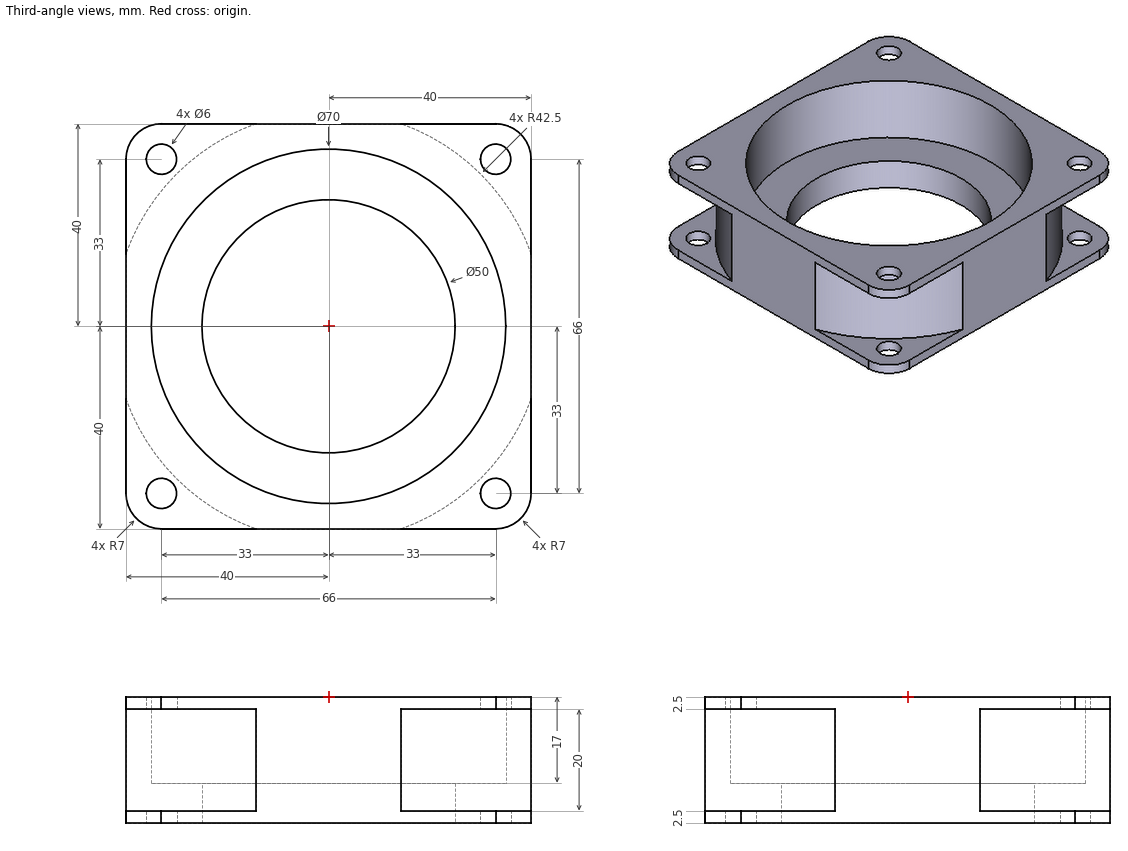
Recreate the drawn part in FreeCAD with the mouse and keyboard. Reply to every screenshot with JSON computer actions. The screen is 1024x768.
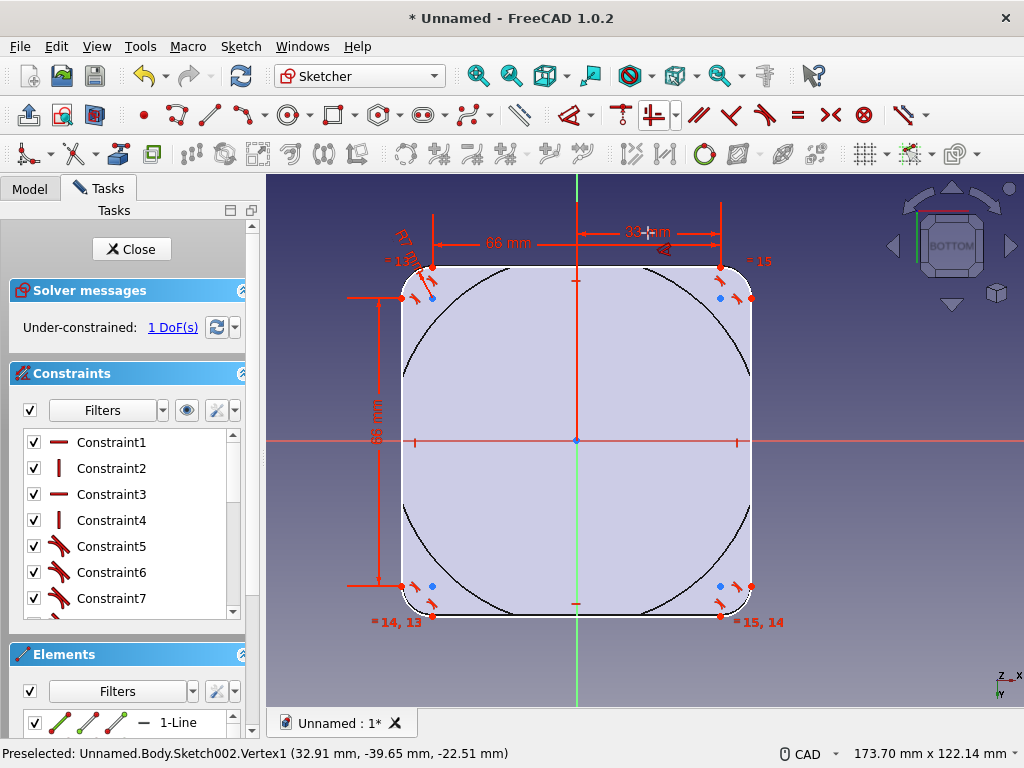
{"action": "left_click", "coordinate": [721, 267]}
{"action": "left_click", "coordinate": [543, 354]}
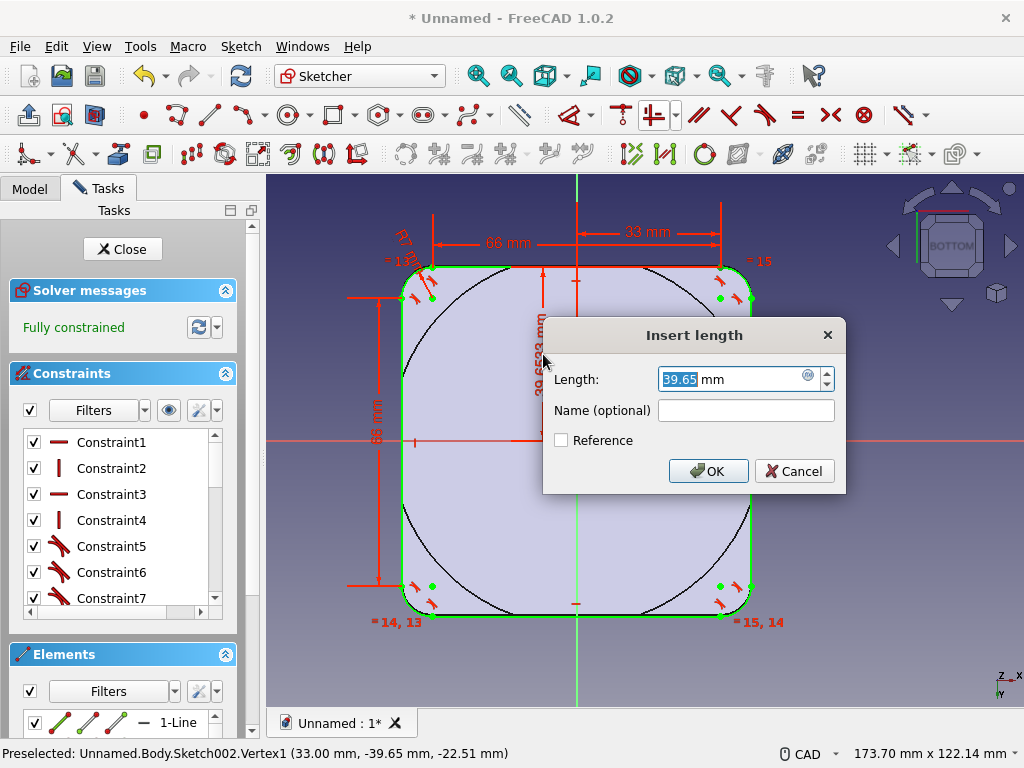
{"action": "type", "text": "40"}
{"action": "key", "text": "Return"}
{"action": "key", "text": "Escape"}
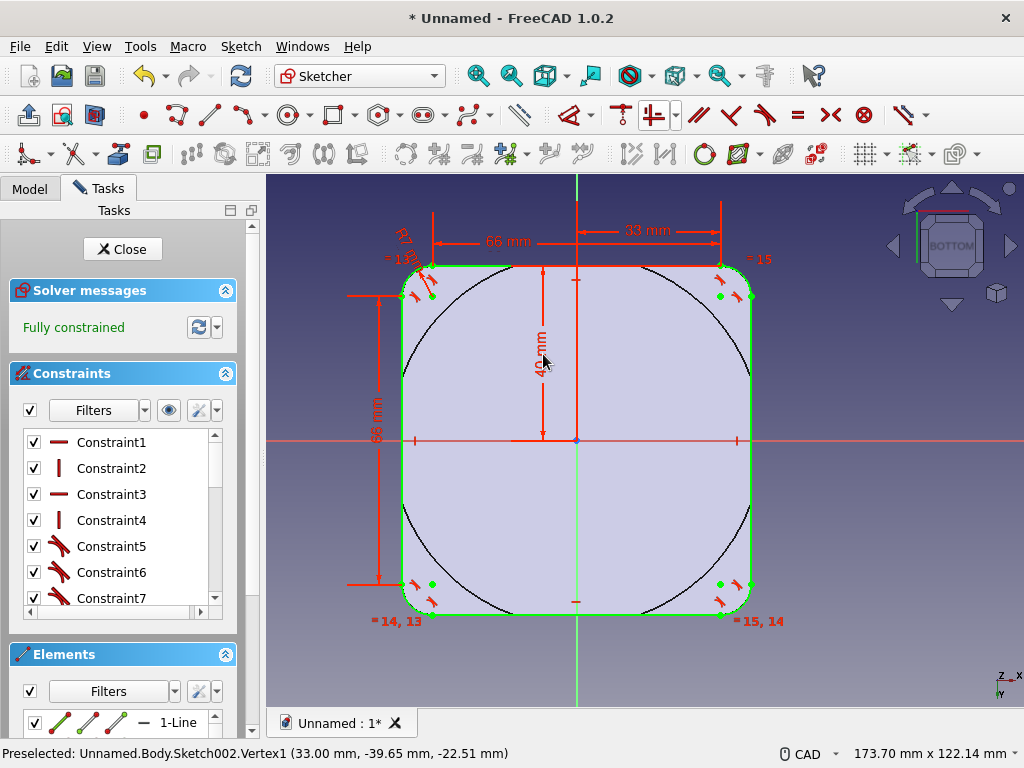
{"action": "left_click", "coordinate": [123, 249]}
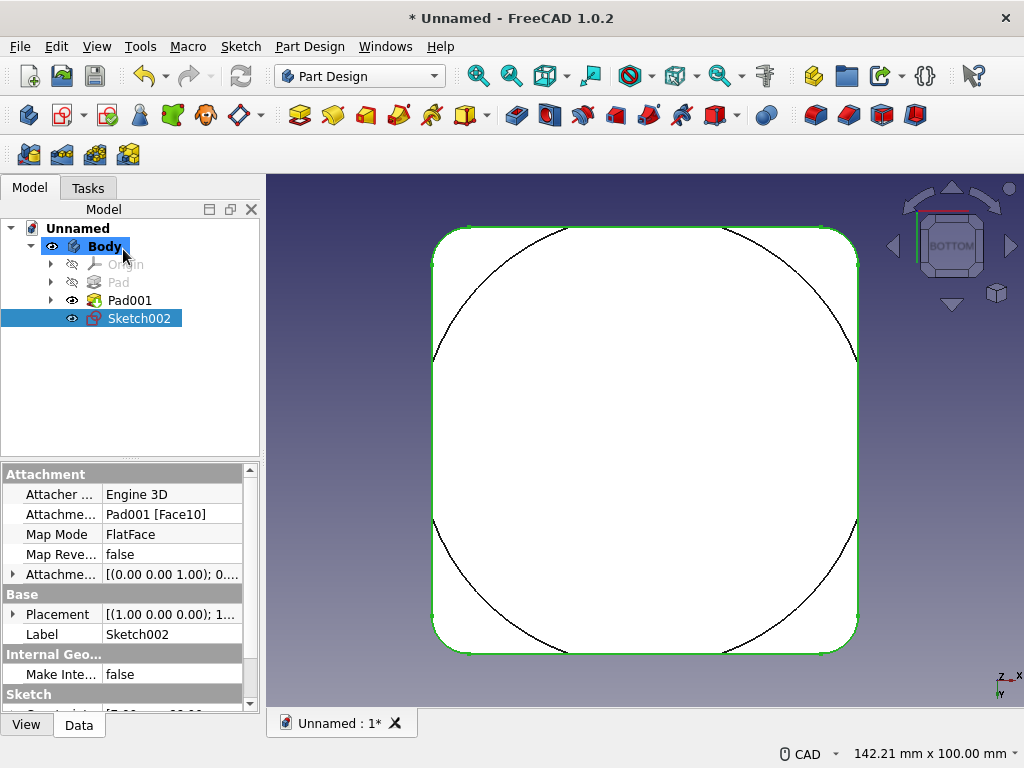
{"action": "left_click", "coordinate": [300, 116]}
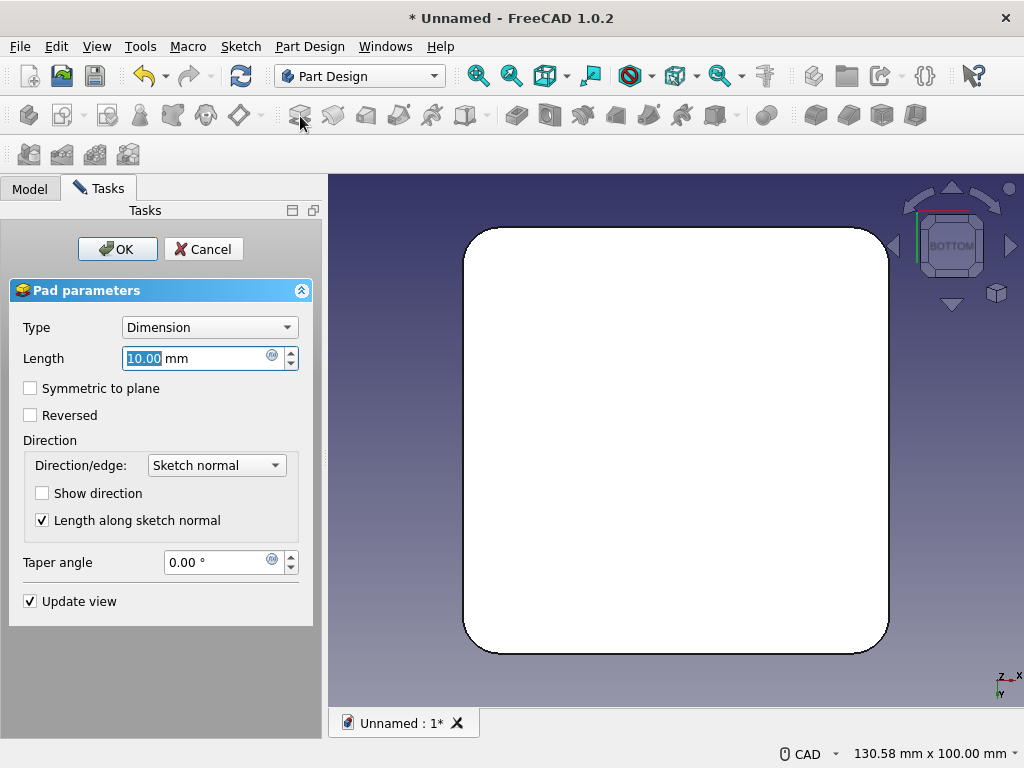
{"action": "type", "text": "2.5"}
{"action": "key", "text": "Tab"}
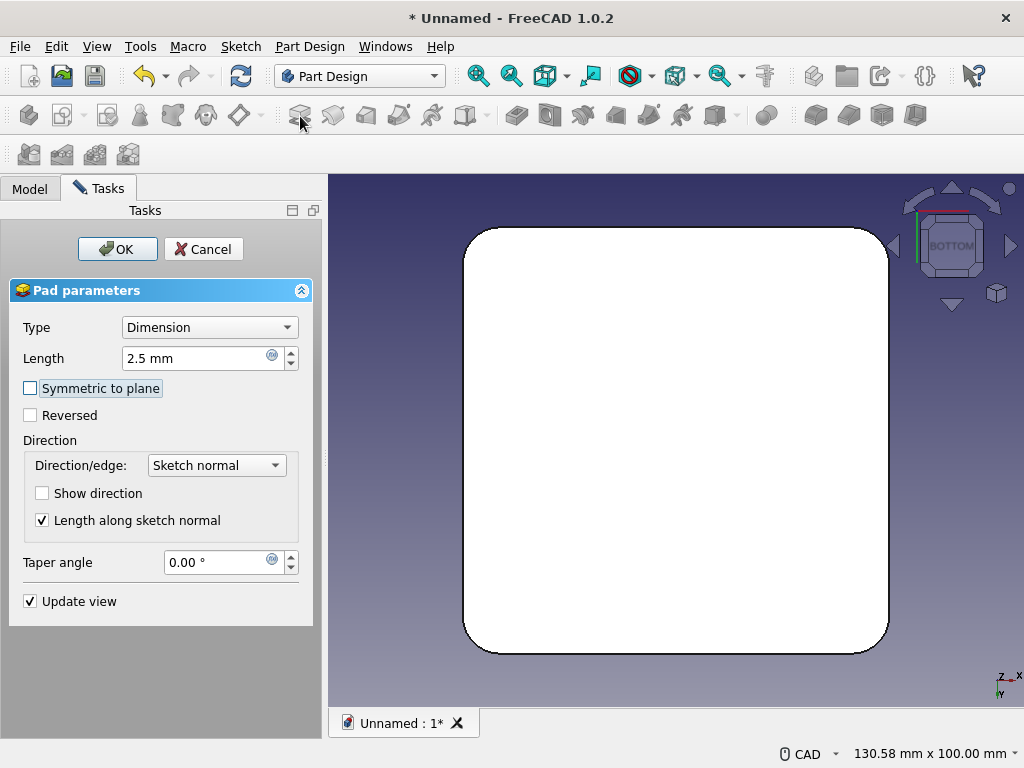
{"action": "left_click", "coordinate": [118, 249]}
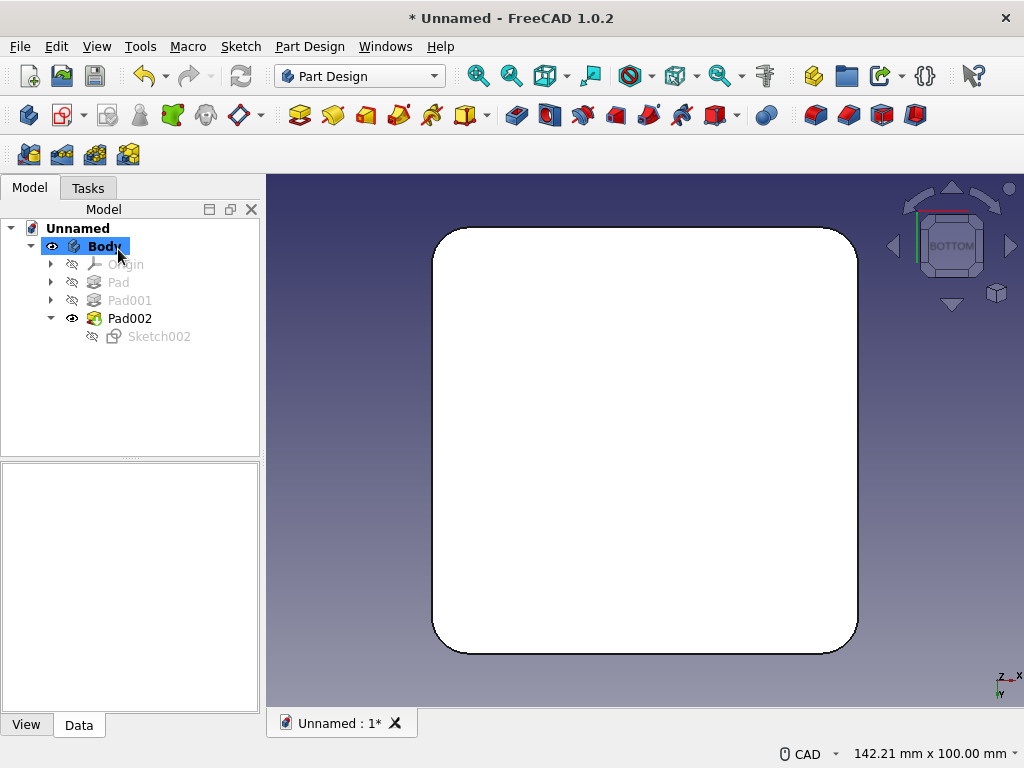
{"action": "key", "text": "0"}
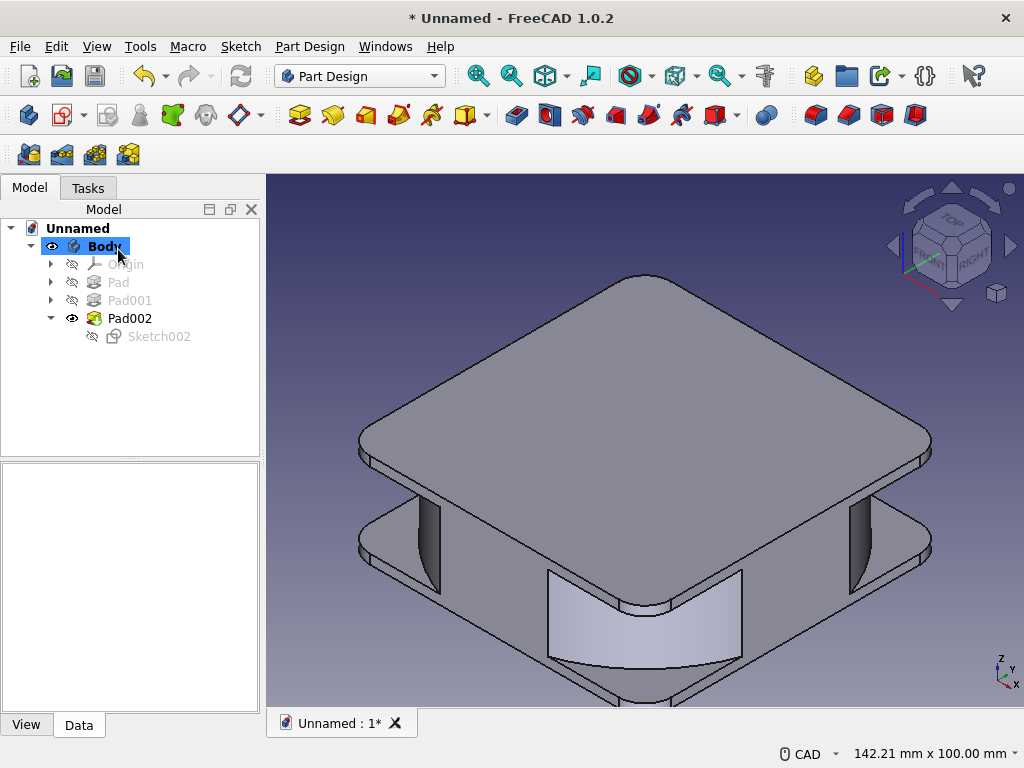
{"action": "left_click", "coordinate": [479, 76]}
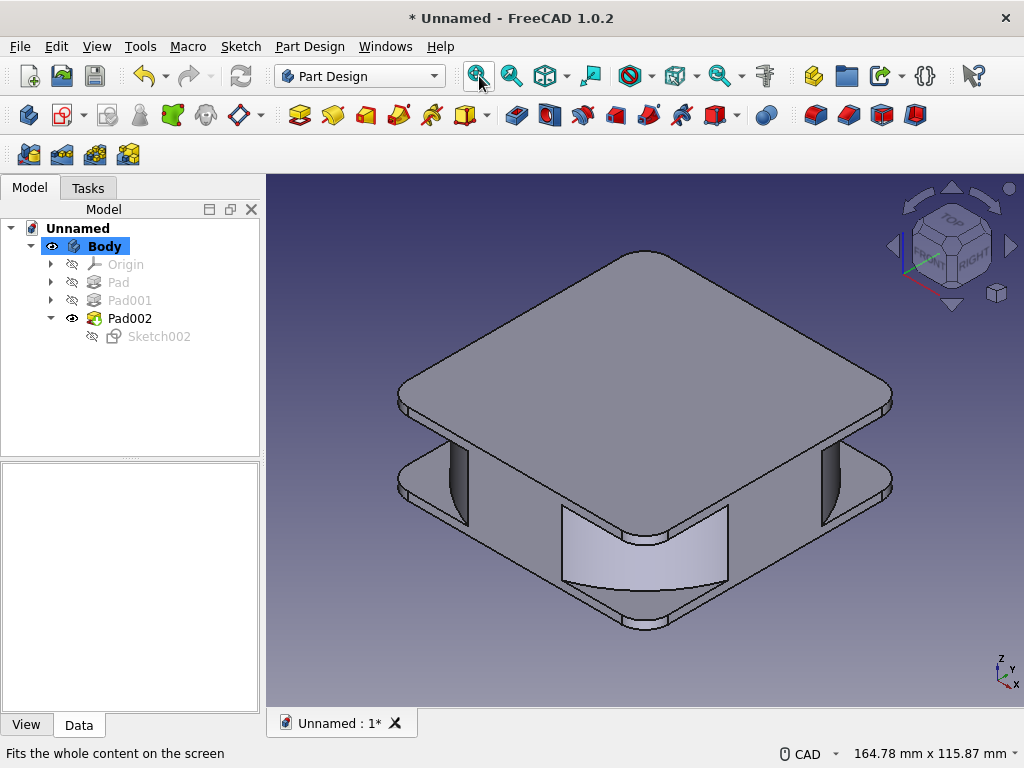
{"action": "left_click", "coordinate": [645, 393]}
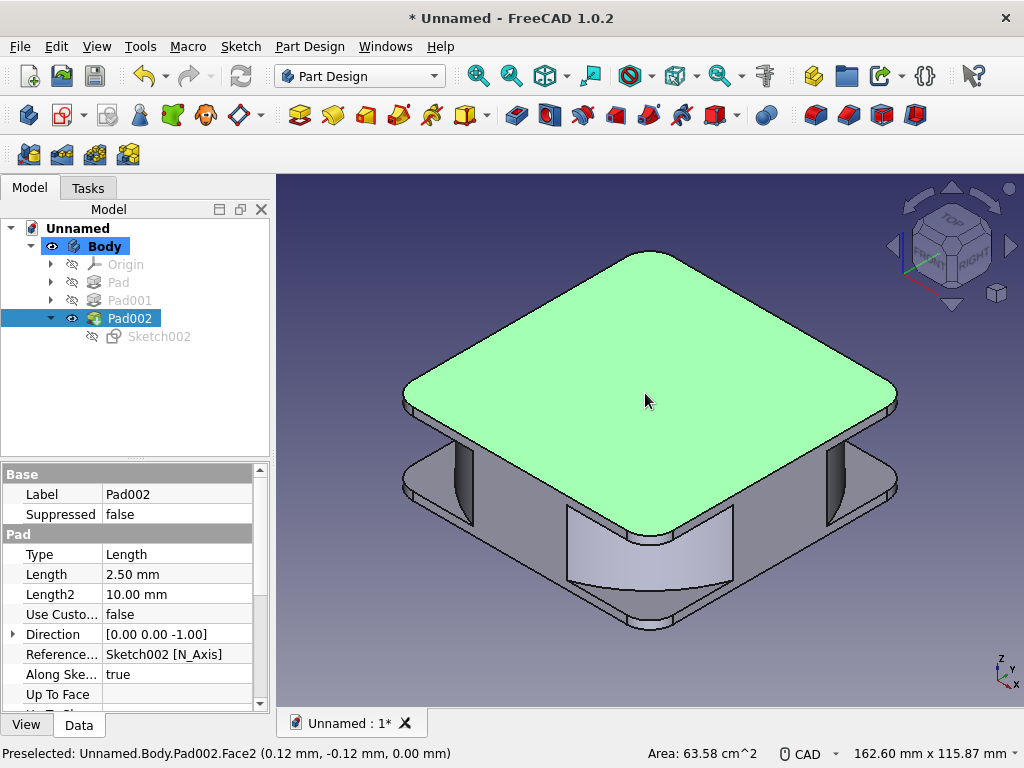
{"action": "left_click", "coordinate": [62, 116]}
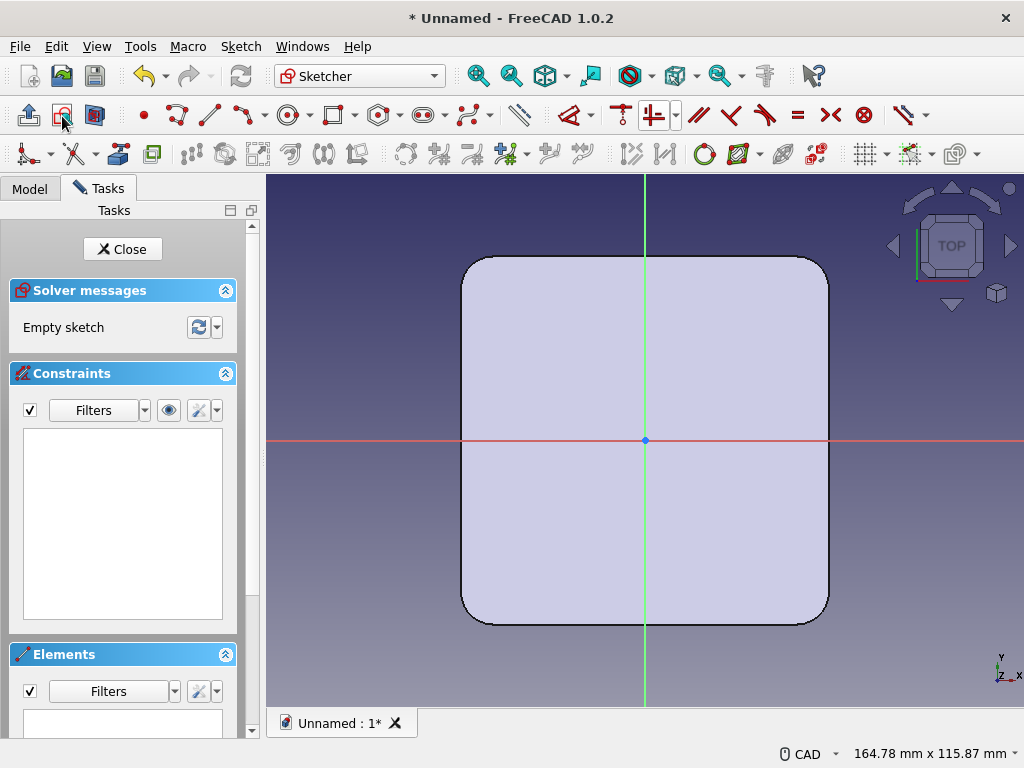
{"action": "left_click", "coordinate": [288, 116]}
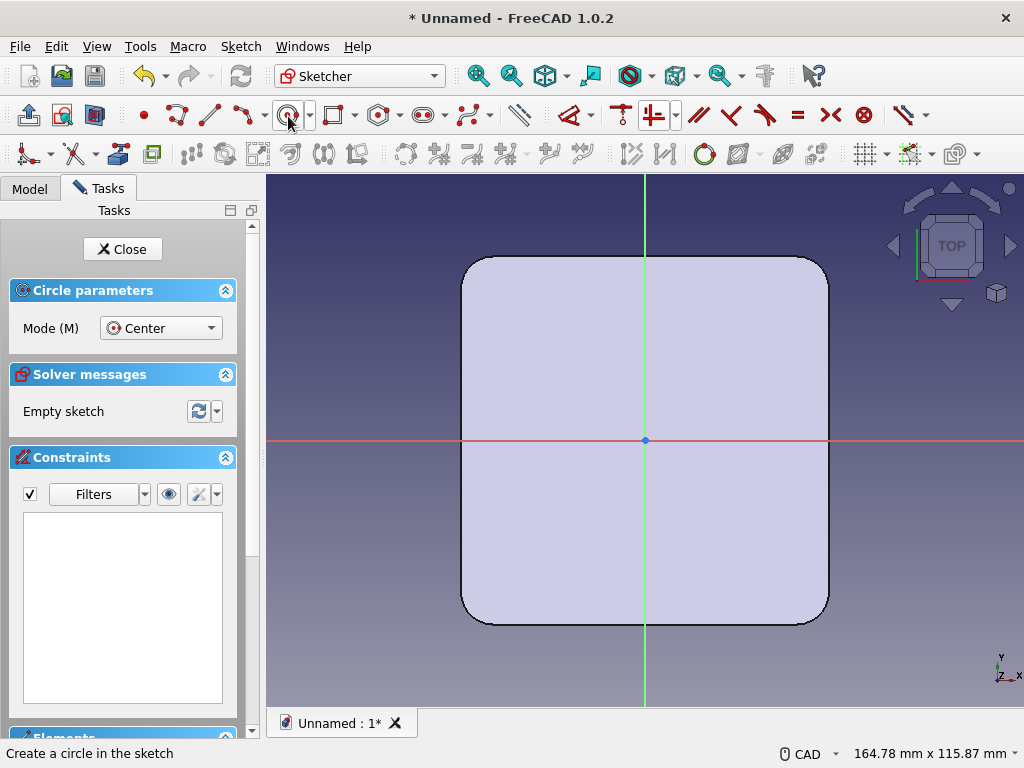
{"action": "scroll", "coordinate": [493, 289], "scroll_direction": "up", "scroll_amount": 3}